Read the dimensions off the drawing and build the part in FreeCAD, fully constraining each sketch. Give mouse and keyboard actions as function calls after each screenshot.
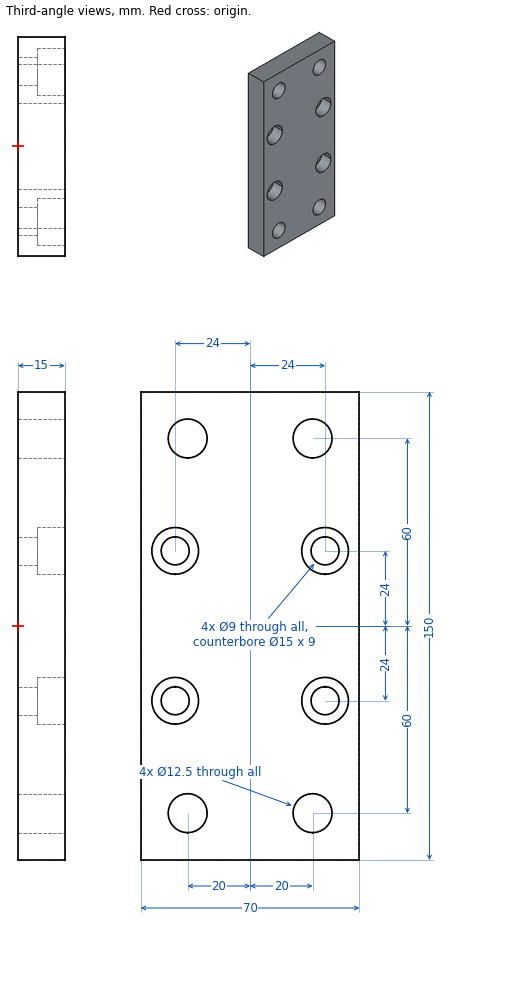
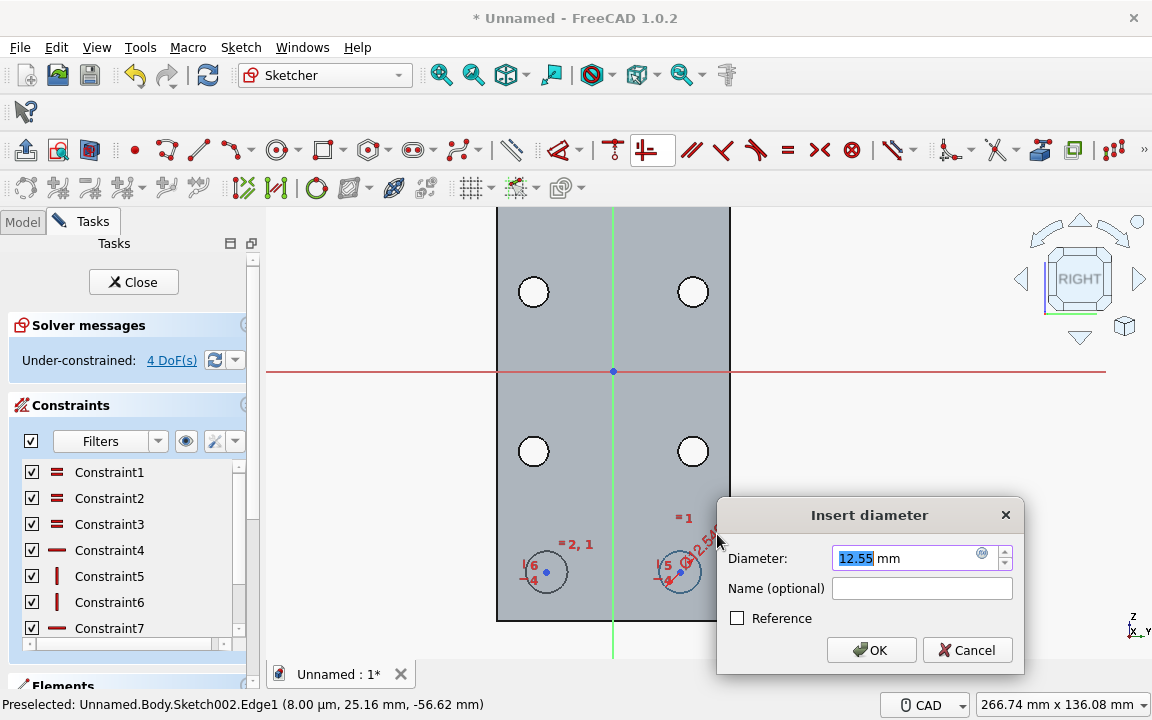
text(12.5)
key(Return)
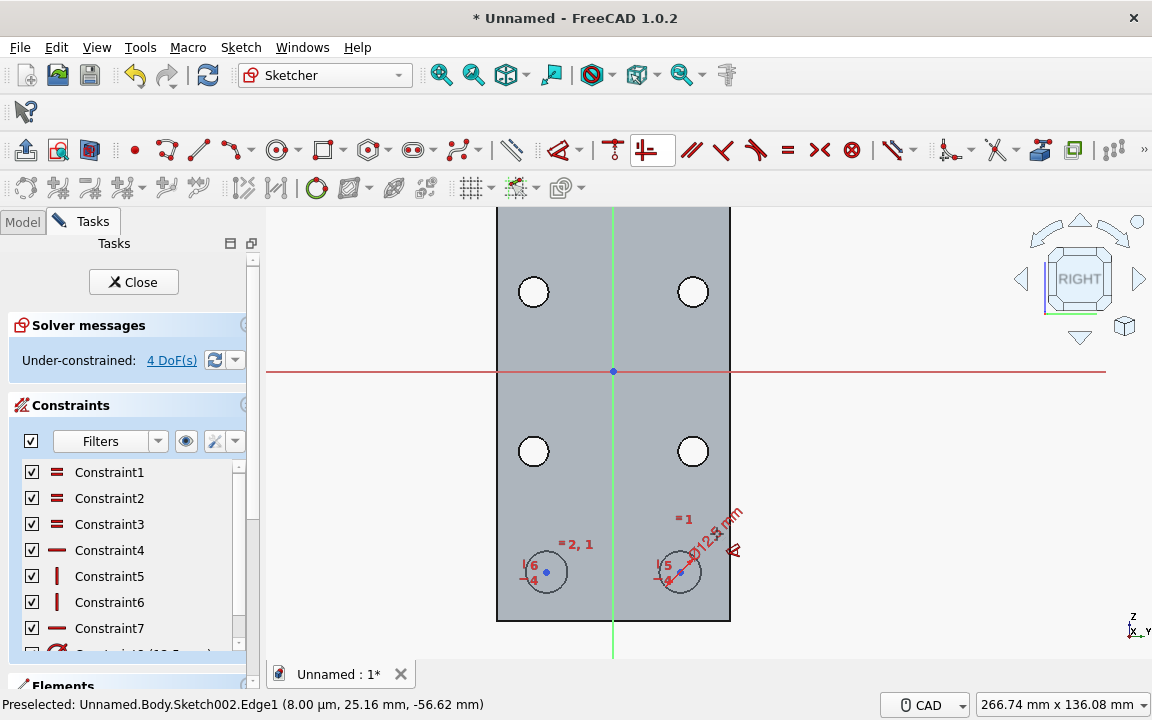
click(680, 572)
click(647, 606)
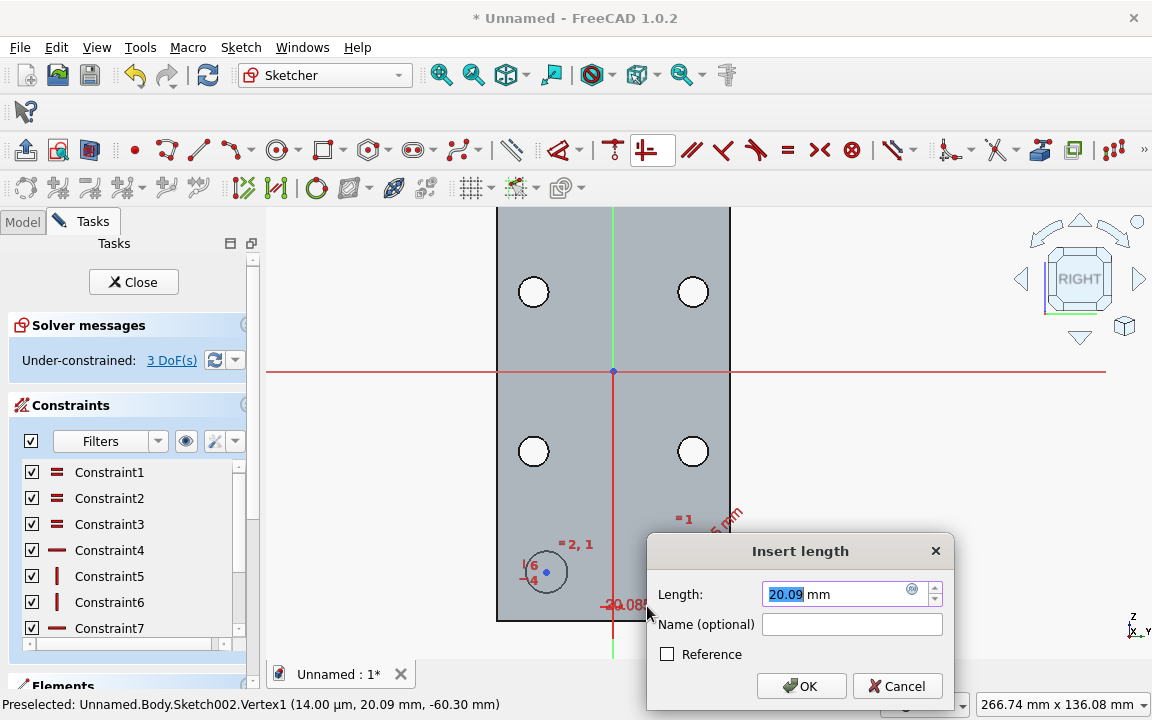
text(20)
key(Return)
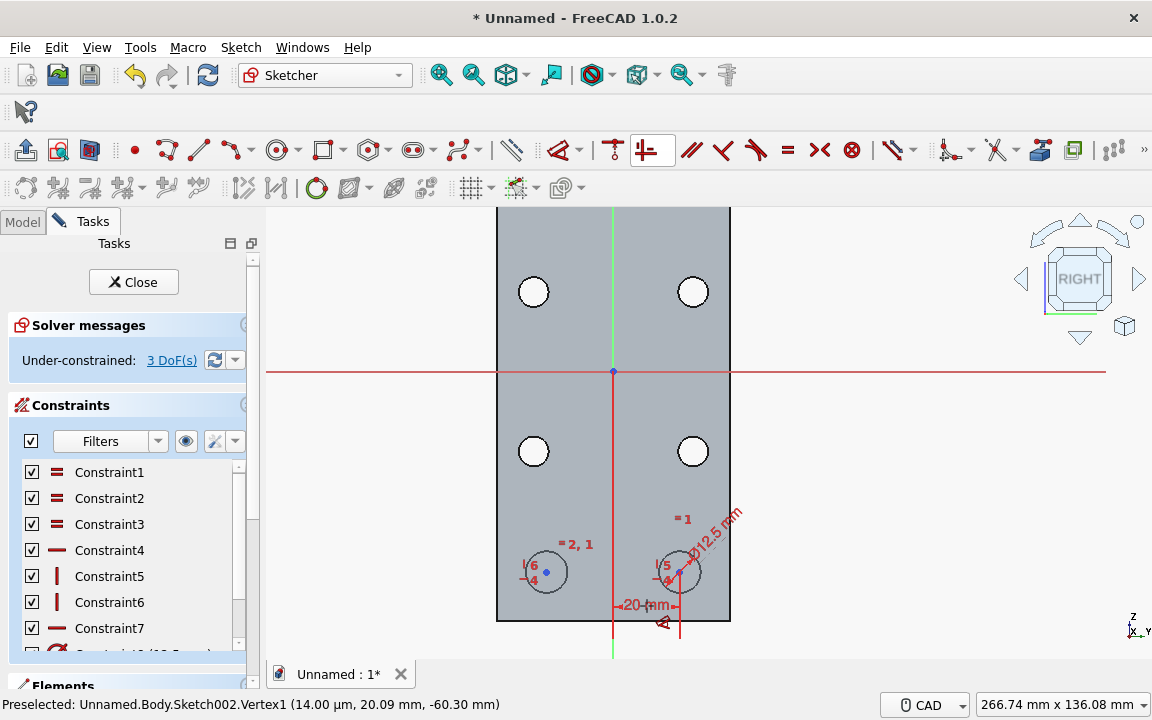
click(680, 572)
click(714, 472)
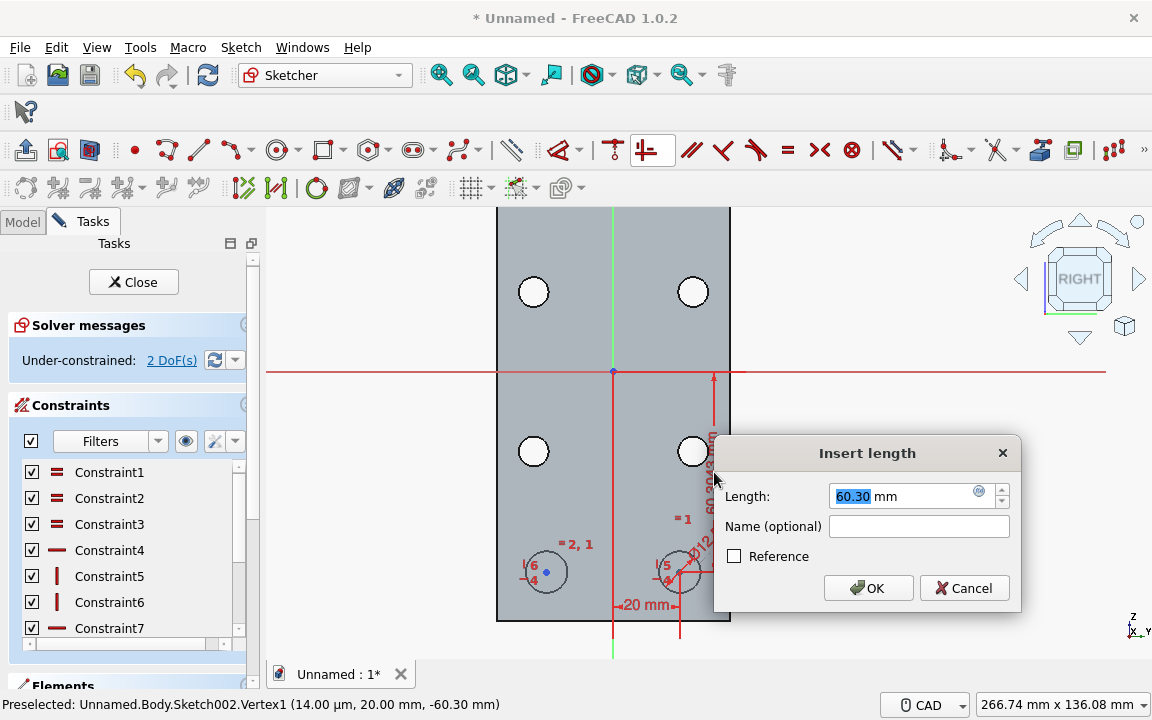
text(60)
key(Return)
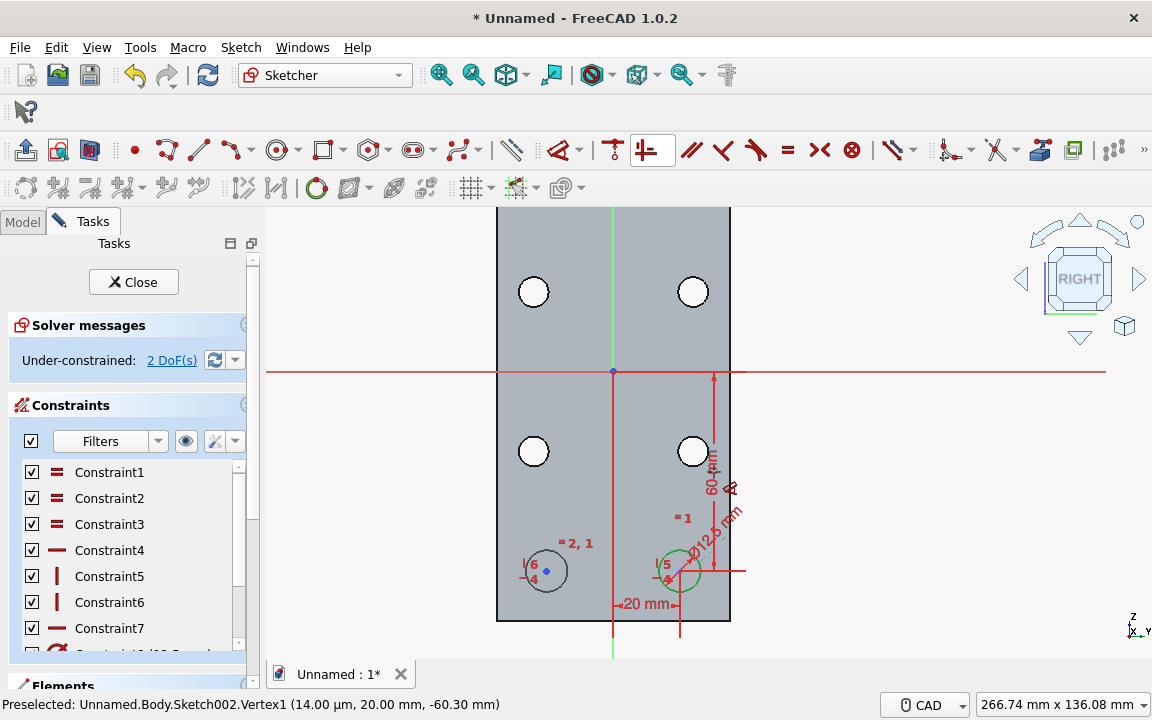
click(547, 571)
click(565, 605)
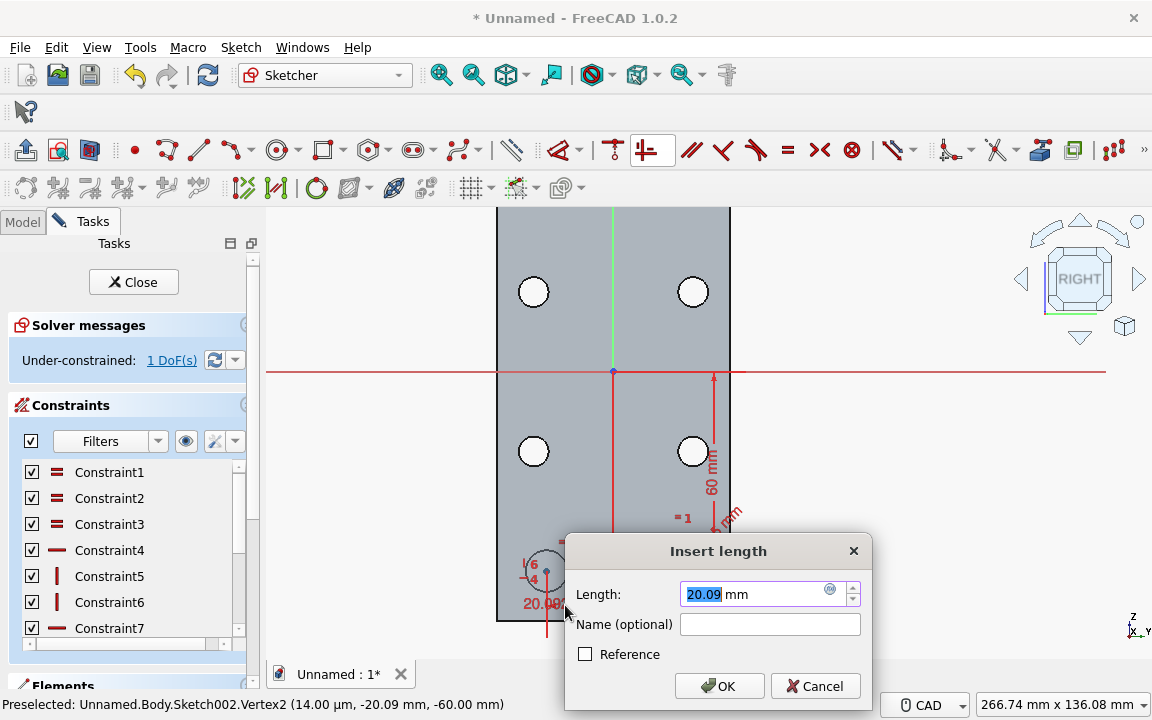
text(20)
key(Return)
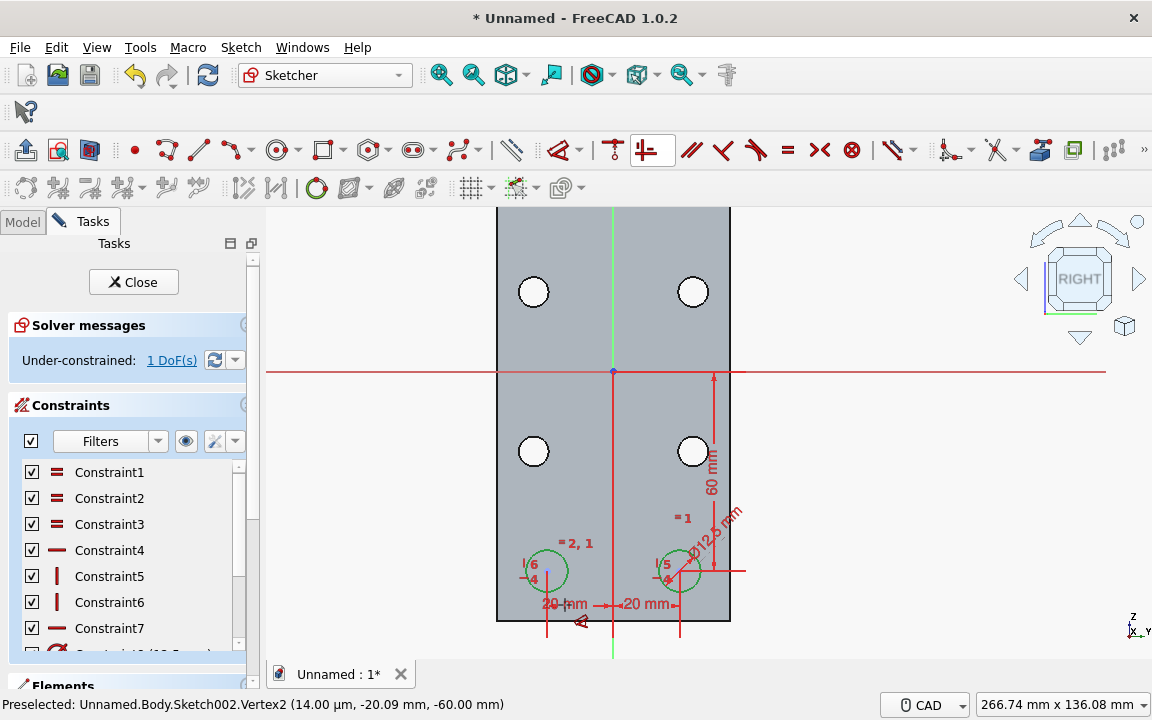
scroll(696, 558, down, 2)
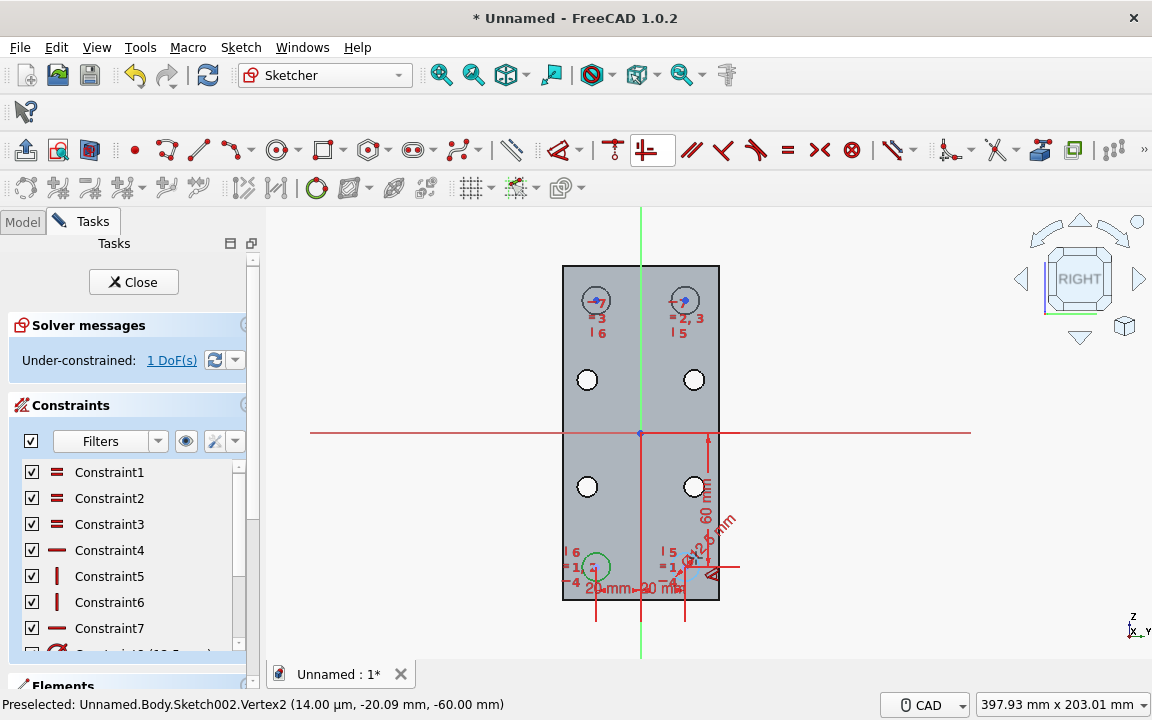
click(685, 301)
click(719, 367)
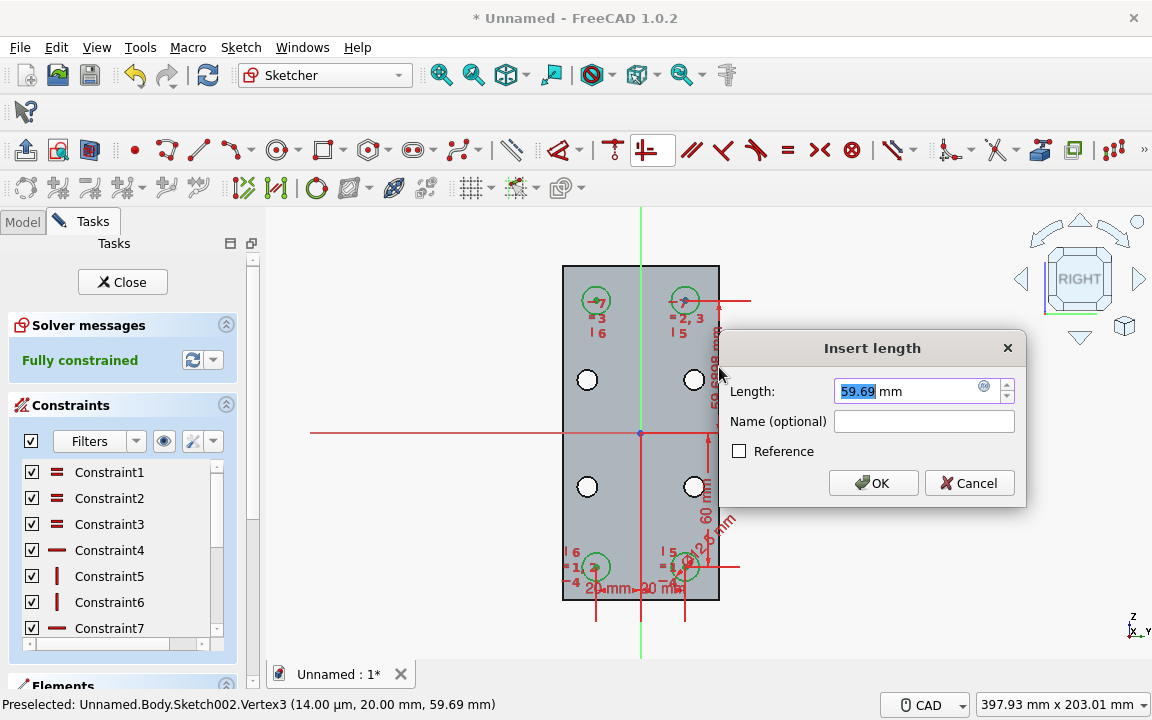
text(60)
key(Return)
key(Escape)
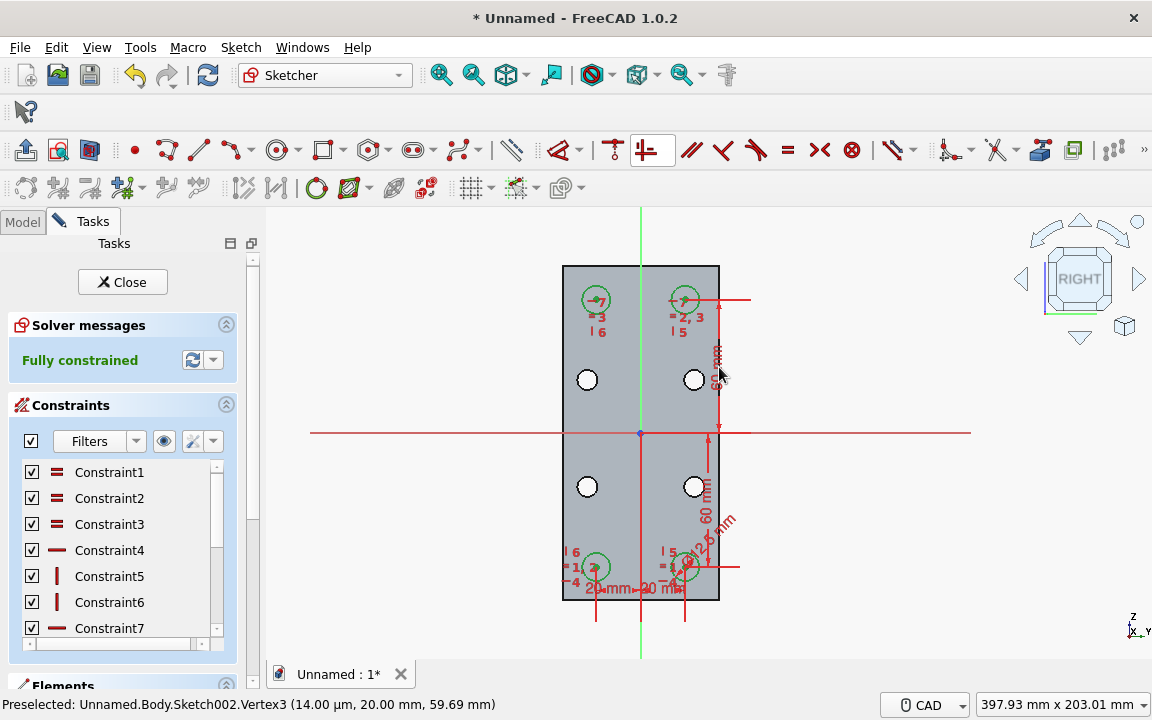
click(123, 282)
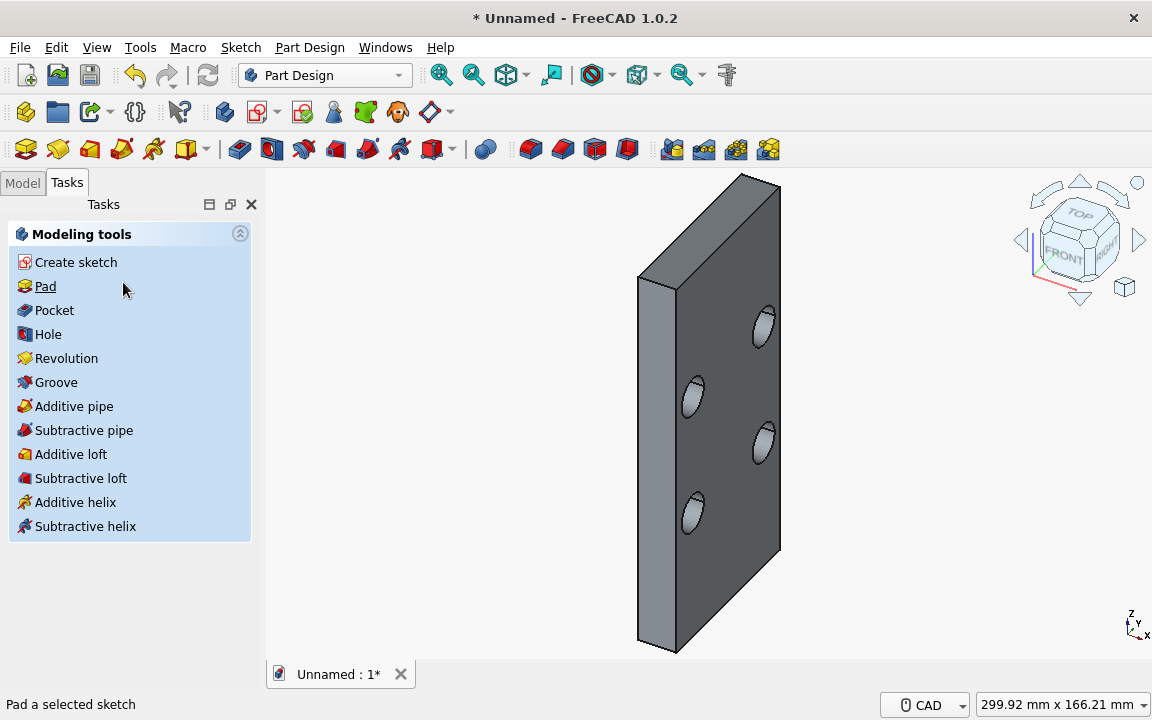
click(272, 150)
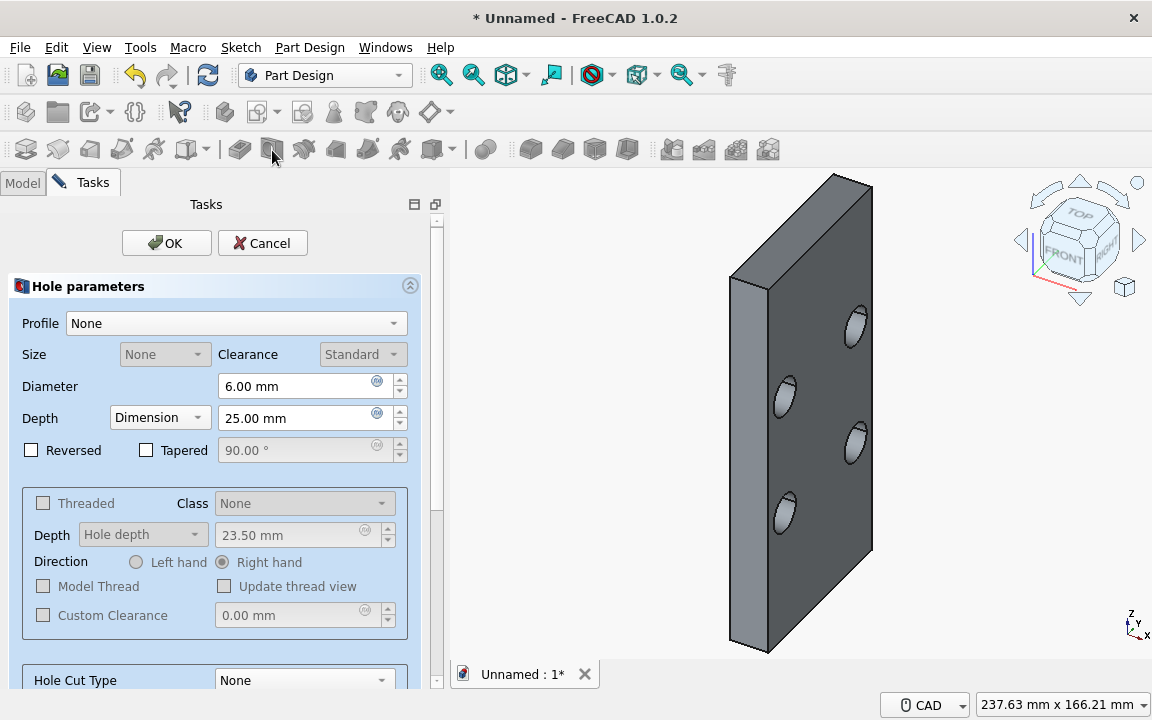
triple_click(305, 386)